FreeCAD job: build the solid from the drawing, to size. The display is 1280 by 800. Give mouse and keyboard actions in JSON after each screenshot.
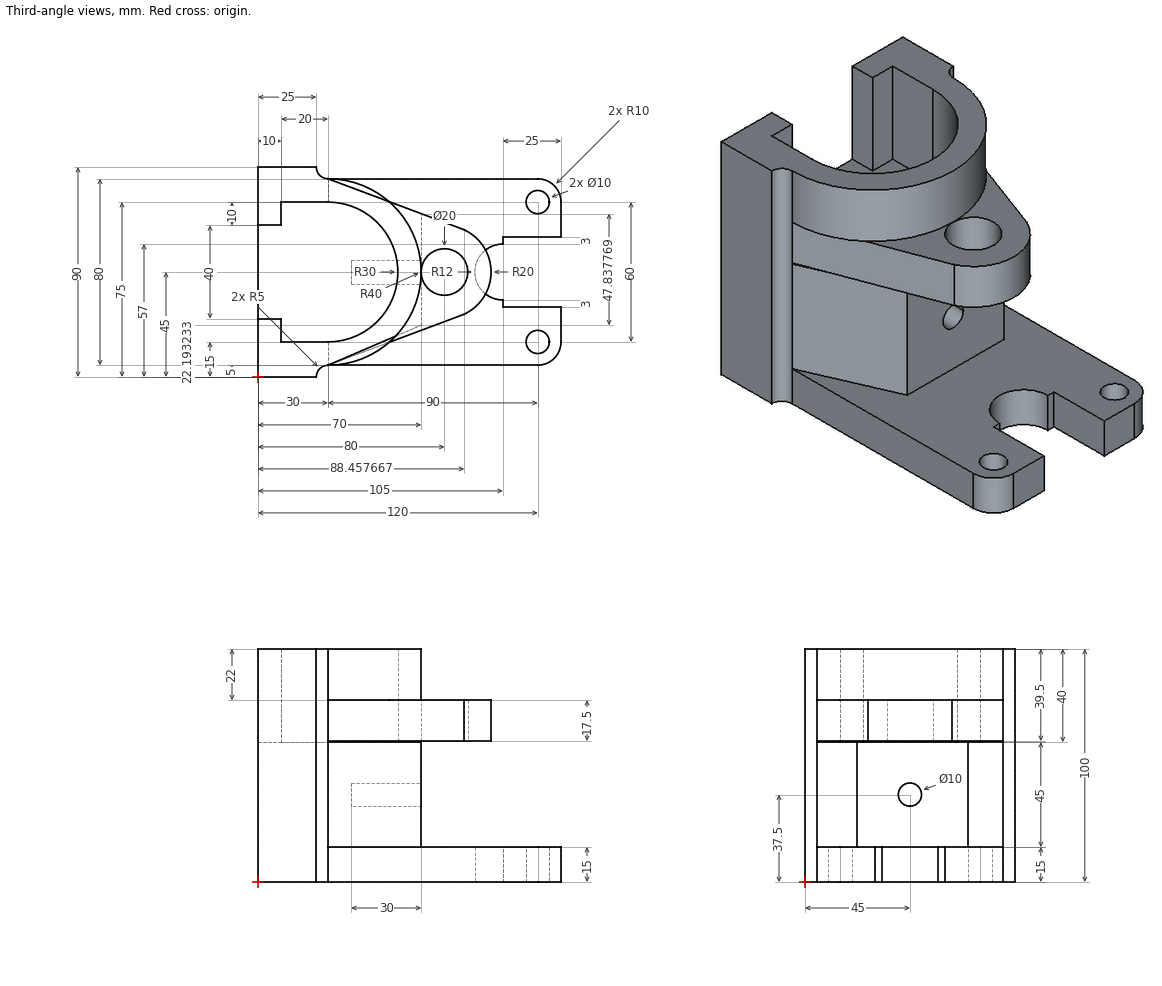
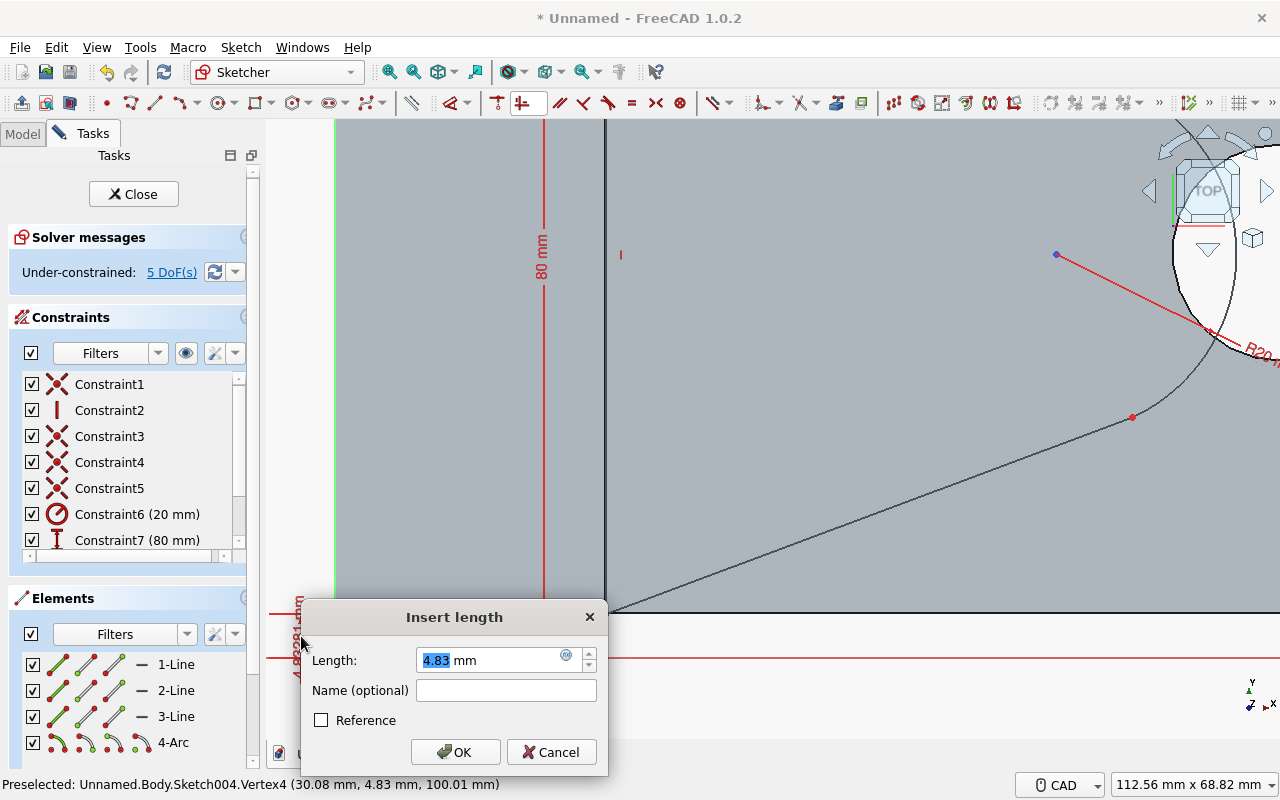
{"action": "type", "text": "5"}
{"action": "key", "text": "Return"}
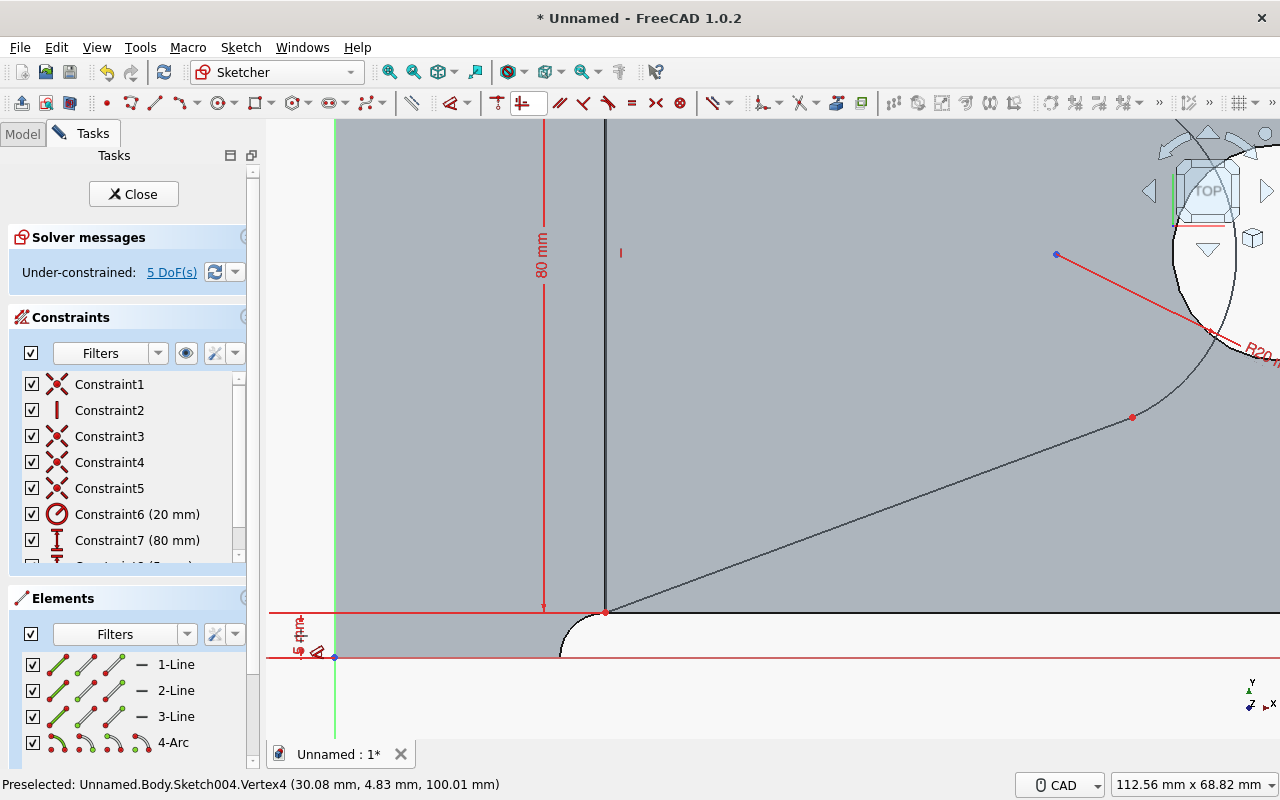
{"action": "scroll", "coordinate": [606, 616], "scroll_direction": "down", "scroll_amount": 3}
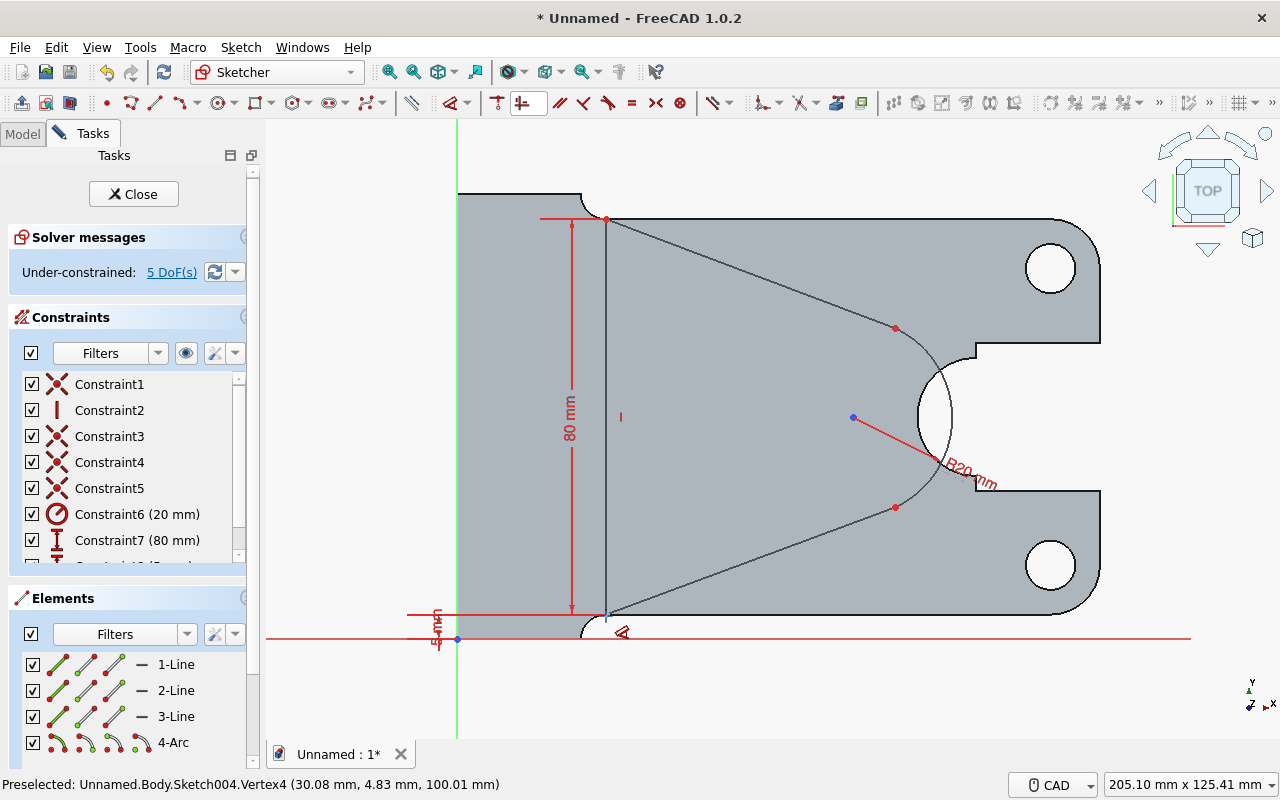
{"action": "left_click", "coordinate": [606, 219]}
{"action": "left_click", "coordinate": [532, 673]}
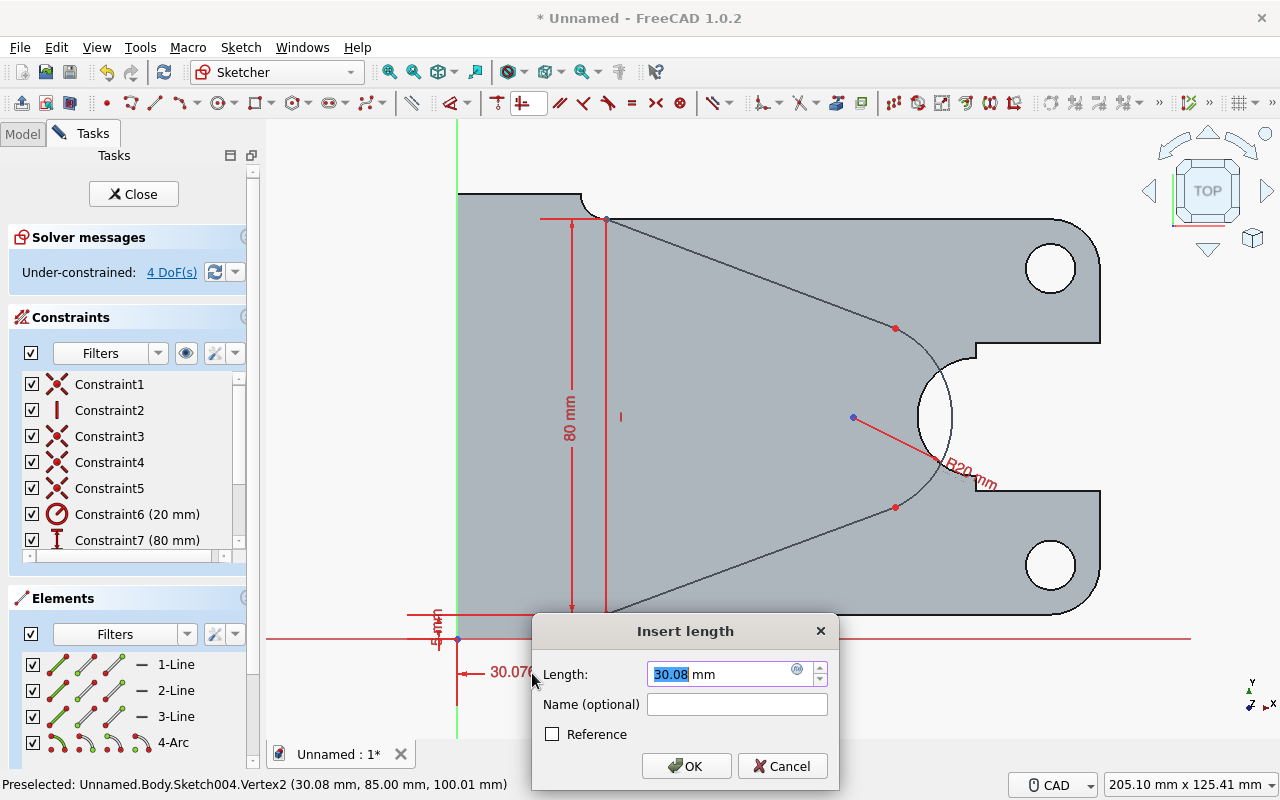
{"action": "type", "text": "30"}
{"action": "key", "text": "Return"}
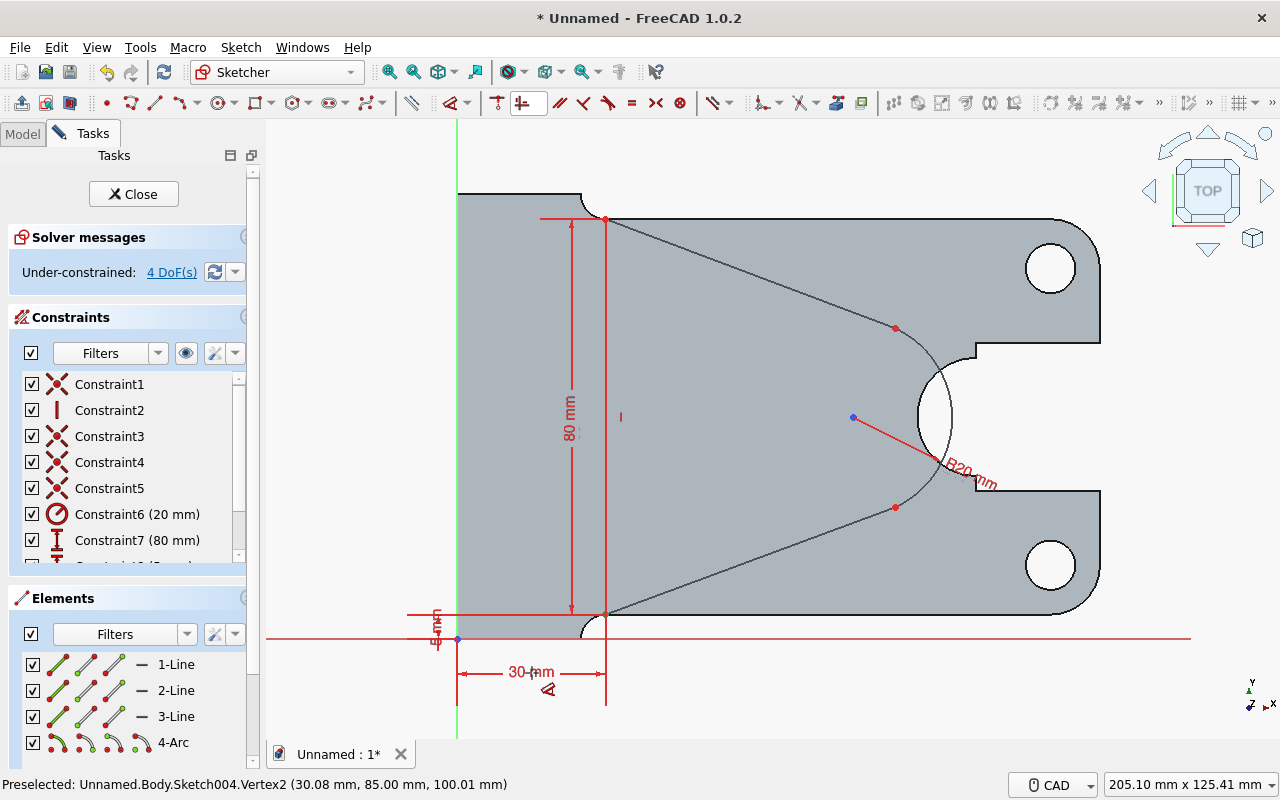
{"action": "left_click", "coordinate": [853, 418]}
{"action": "left_click", "coordinate": [655, 673]}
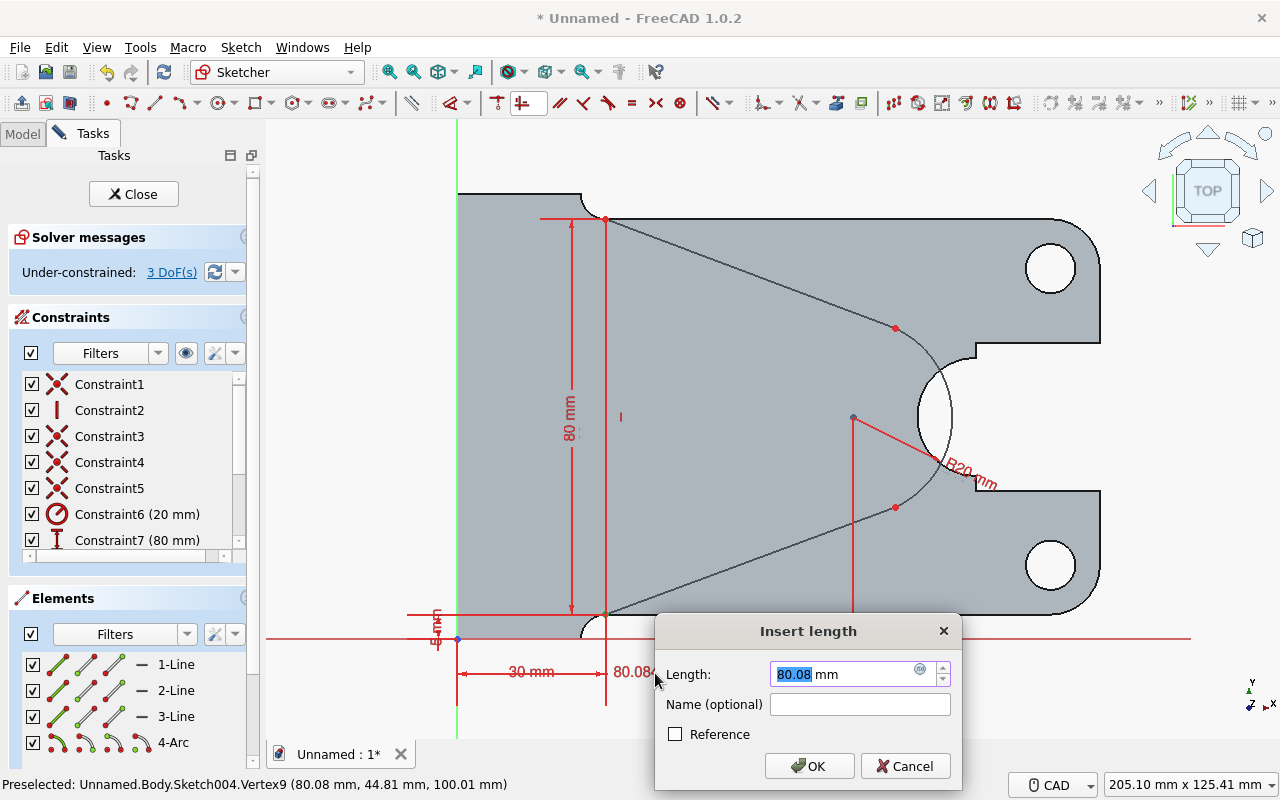
{"action": "type", "text": "80"}
{"action": "key", "text": "Return"}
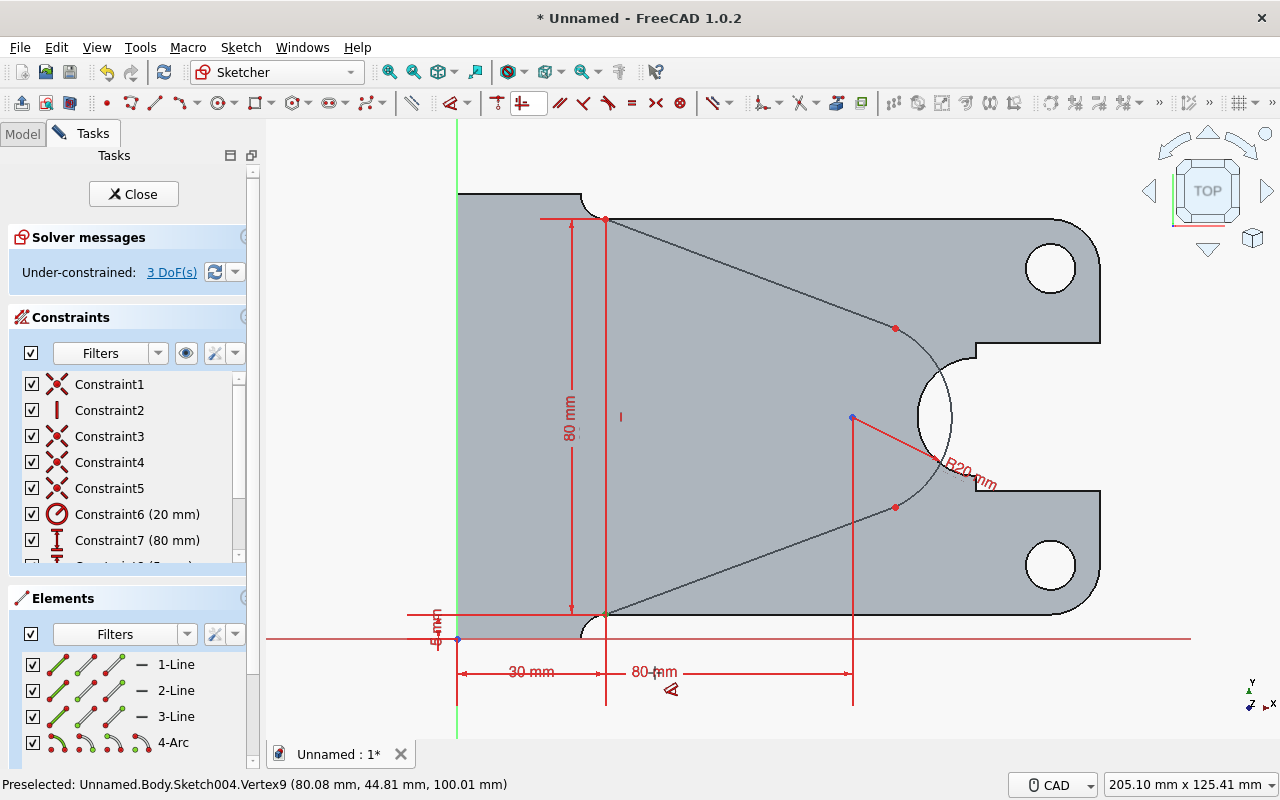
{"action": "left_click", "coordinate": [853, 418]}
{"action": "left_click", "coordinate": [423, 528]}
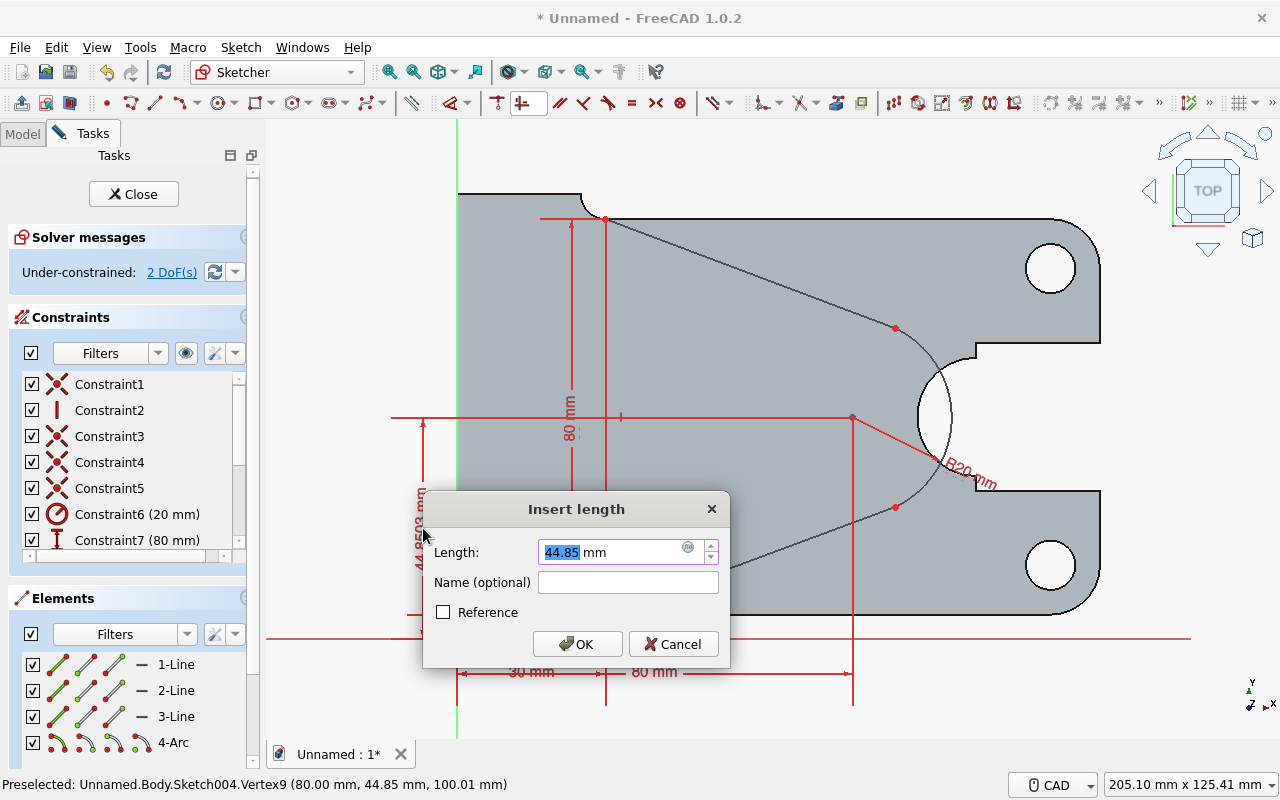
{"action": "type", "text": "45"}
{"action": "key", "text": "Return"}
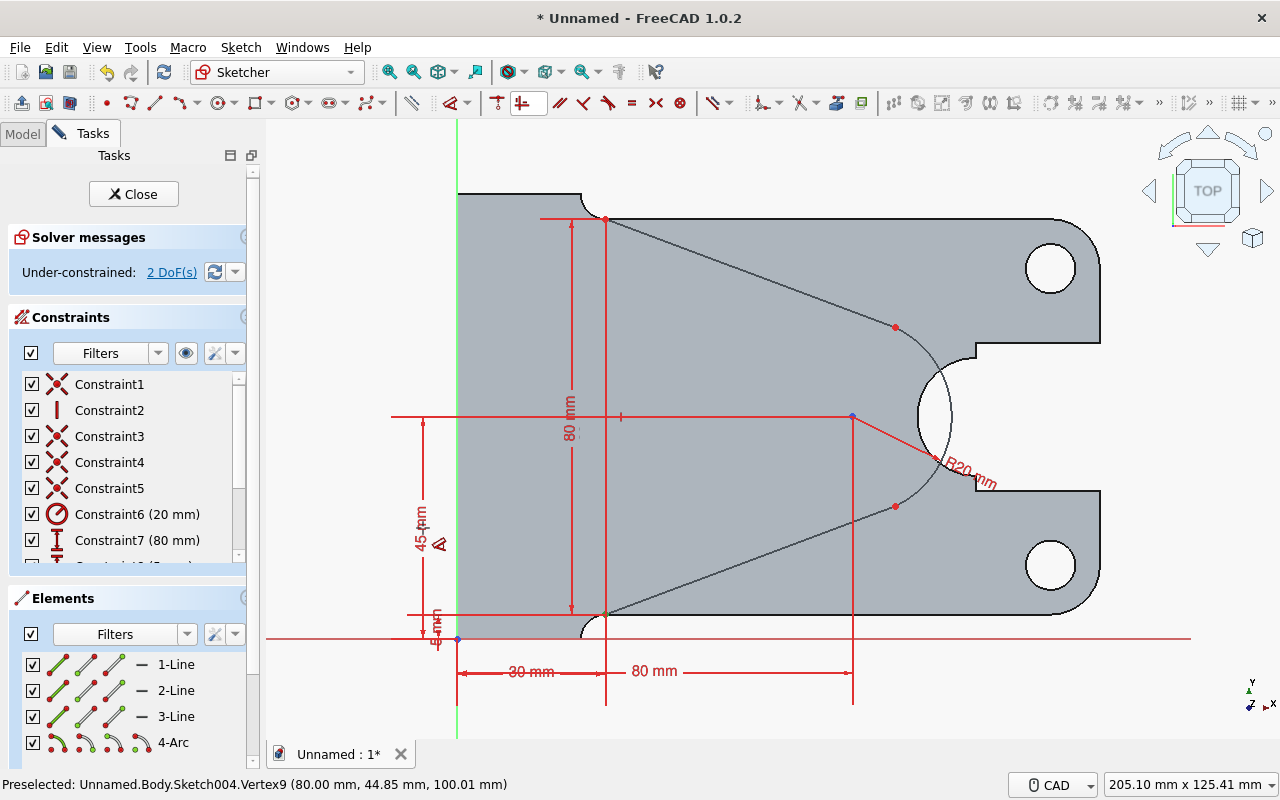
{"action": "left_click", "coordinate": [895, 327]}
{"action": "left_click", "coordinate": [777, 673]}